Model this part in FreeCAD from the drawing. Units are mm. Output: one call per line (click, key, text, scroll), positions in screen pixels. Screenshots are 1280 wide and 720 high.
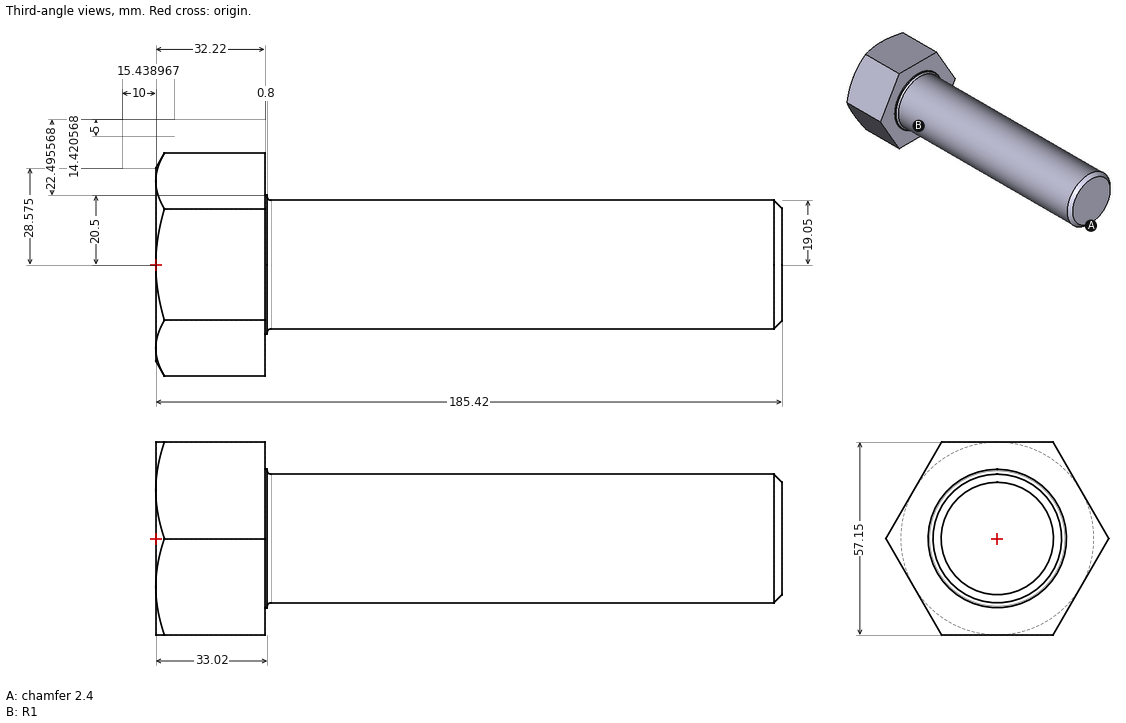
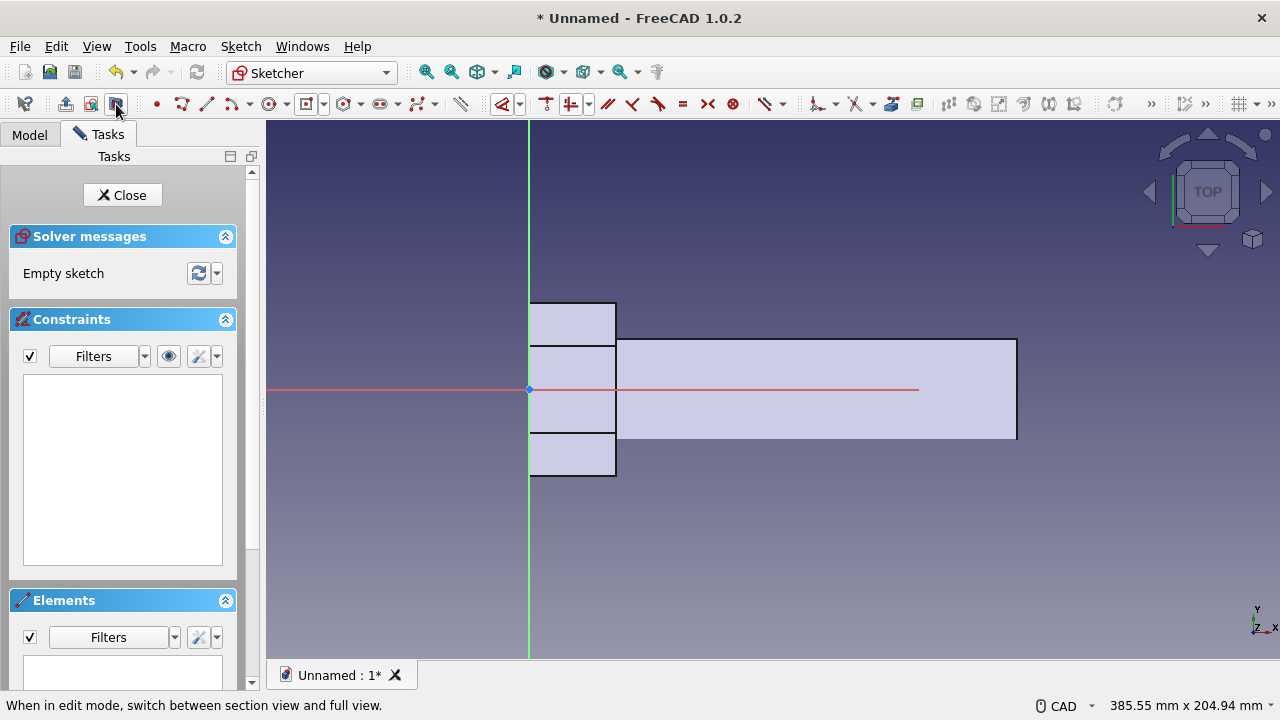
scroll(501, 284, up, 11)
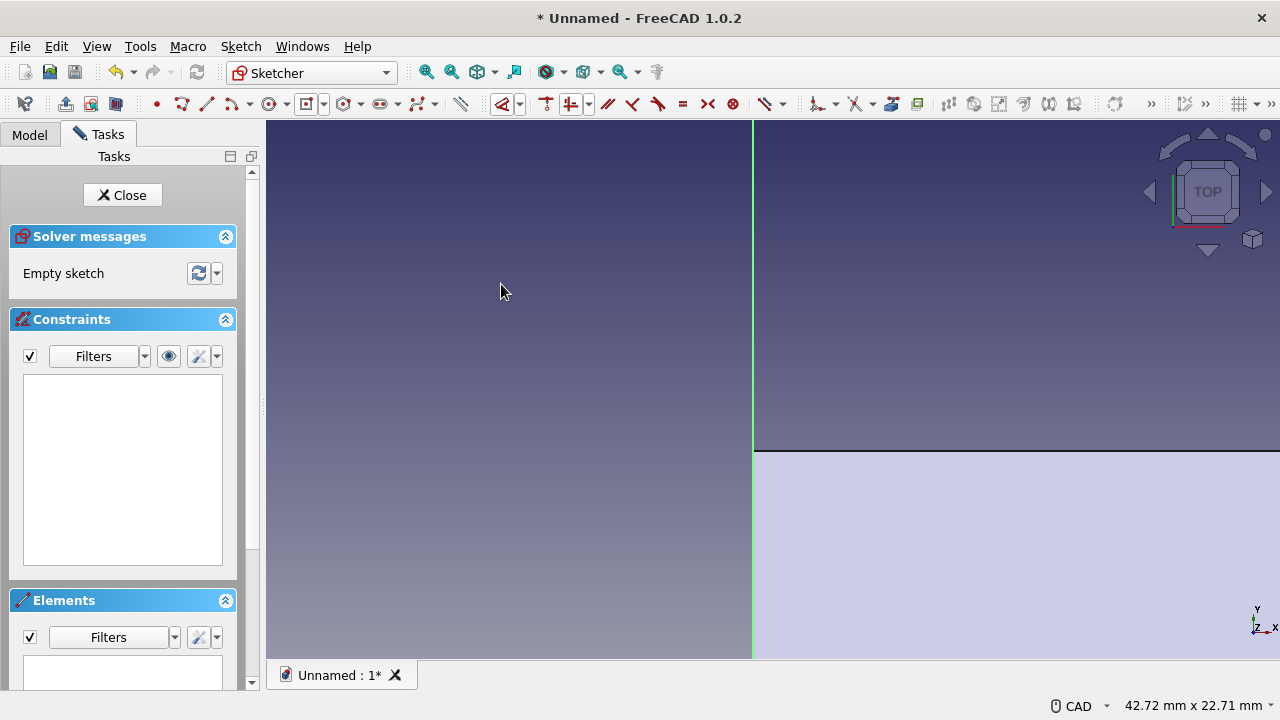
click(182, 104)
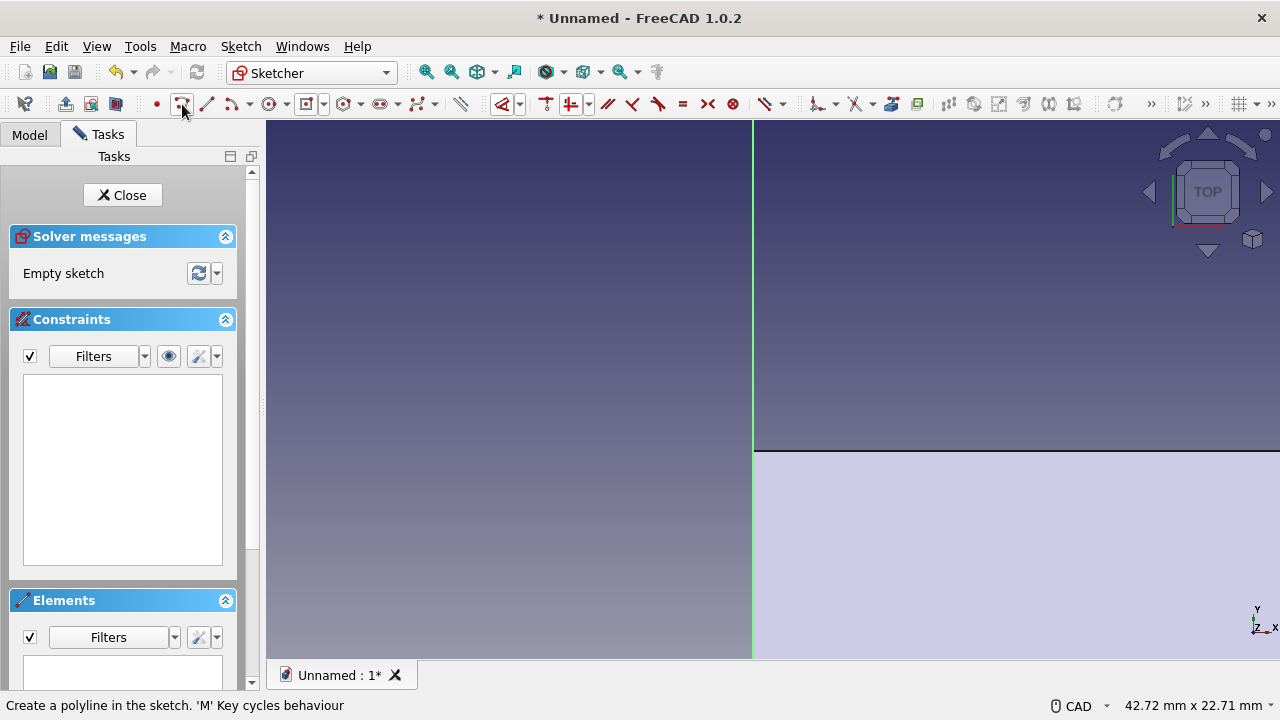
click(753, 555)
click(882, 332)
click(882, 213)
click(516, 213)
click(516, 555)
click(753, 556)
key(Escape)
key(Escape)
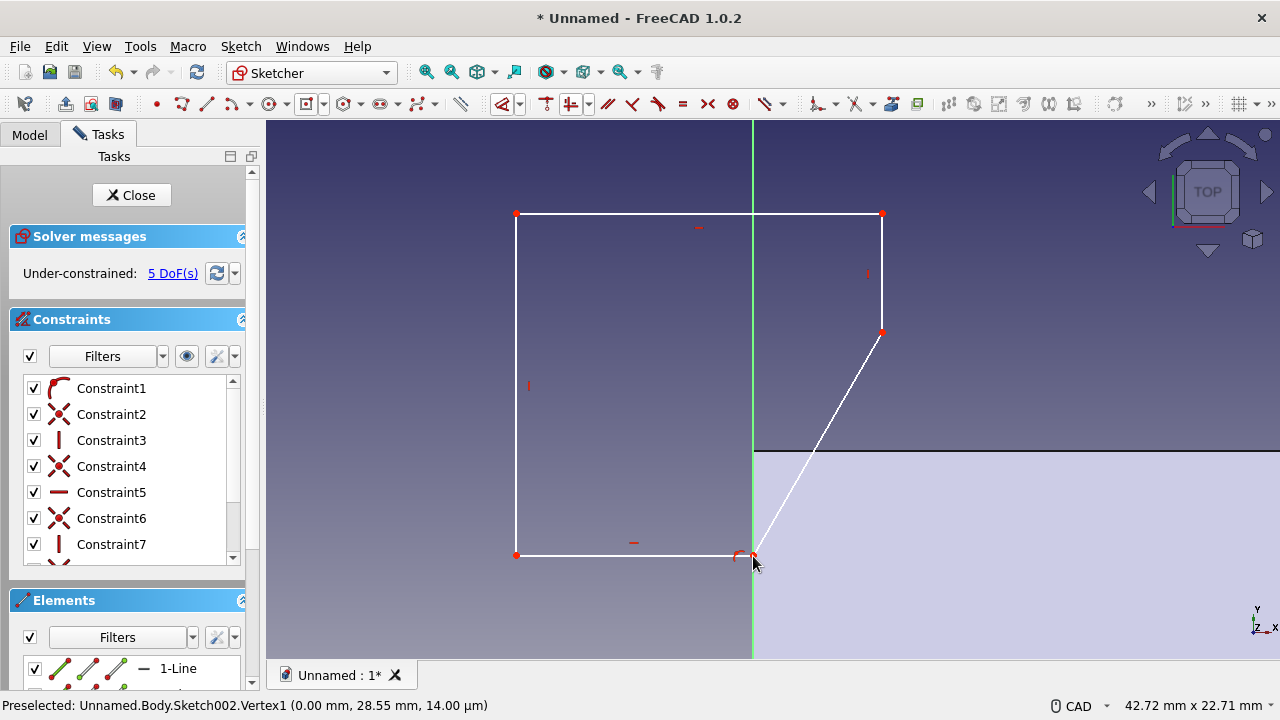
click(882, 297)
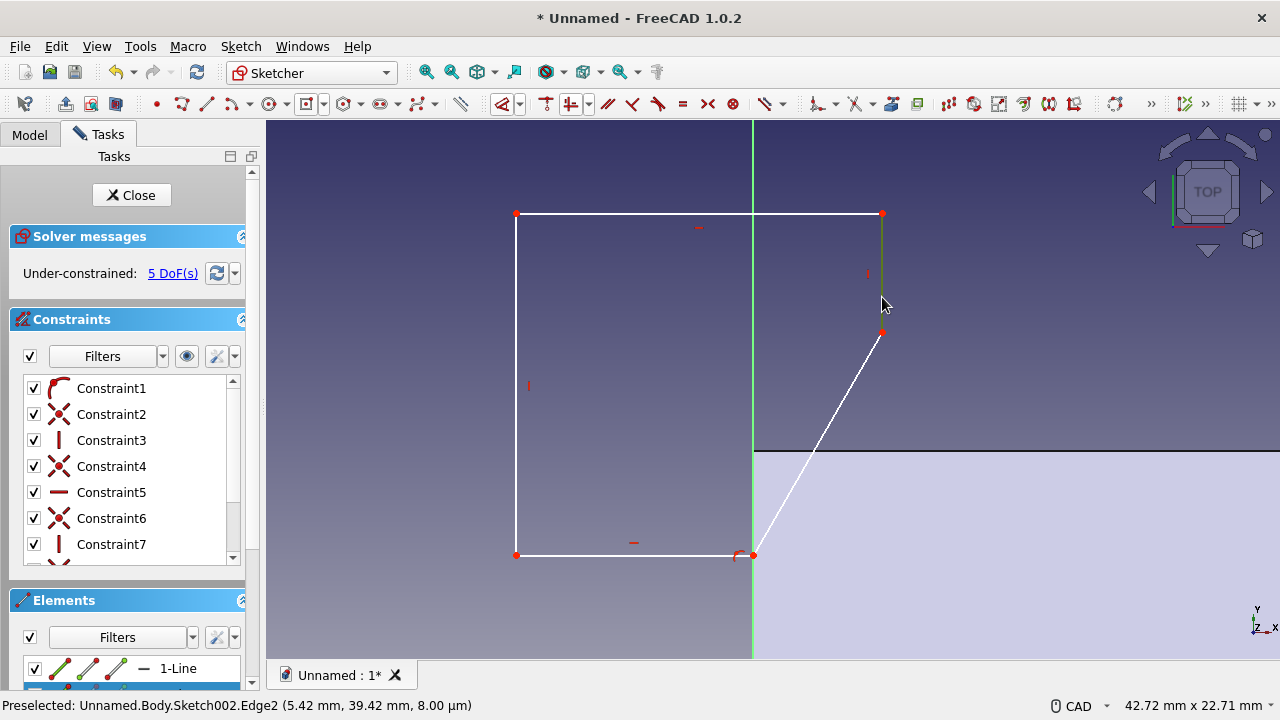
key(i)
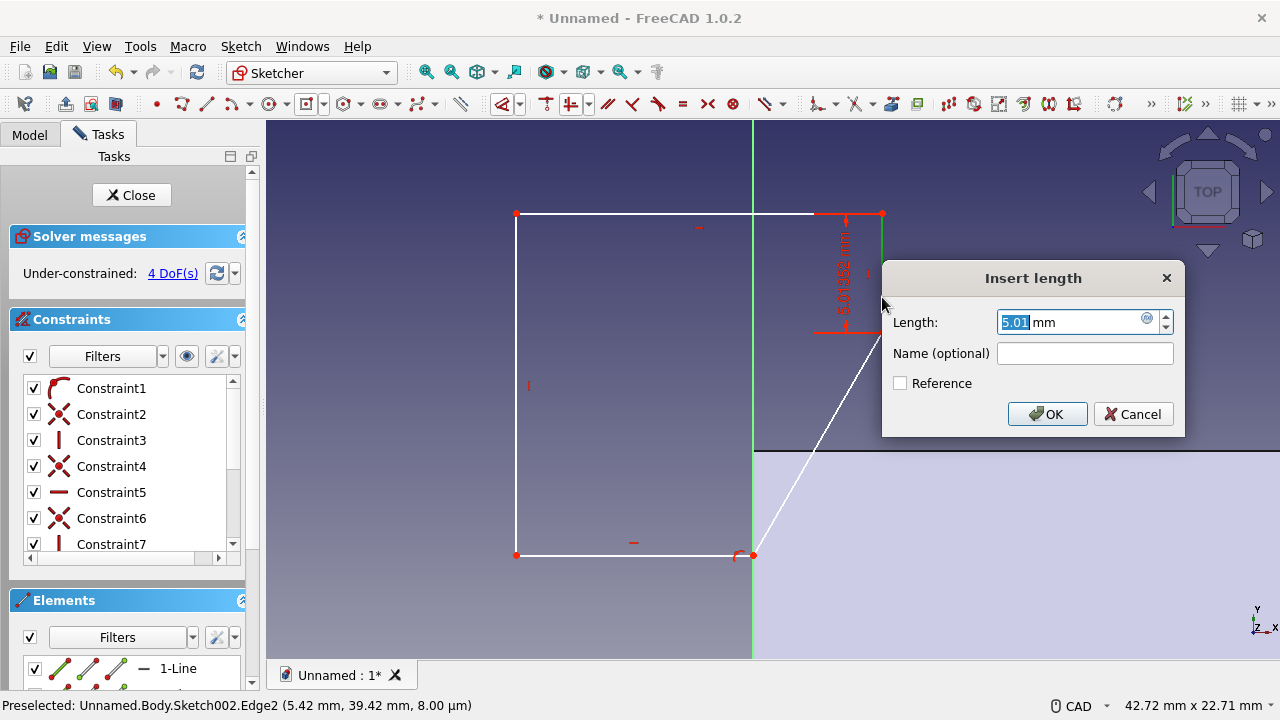
text(5)
key(Return)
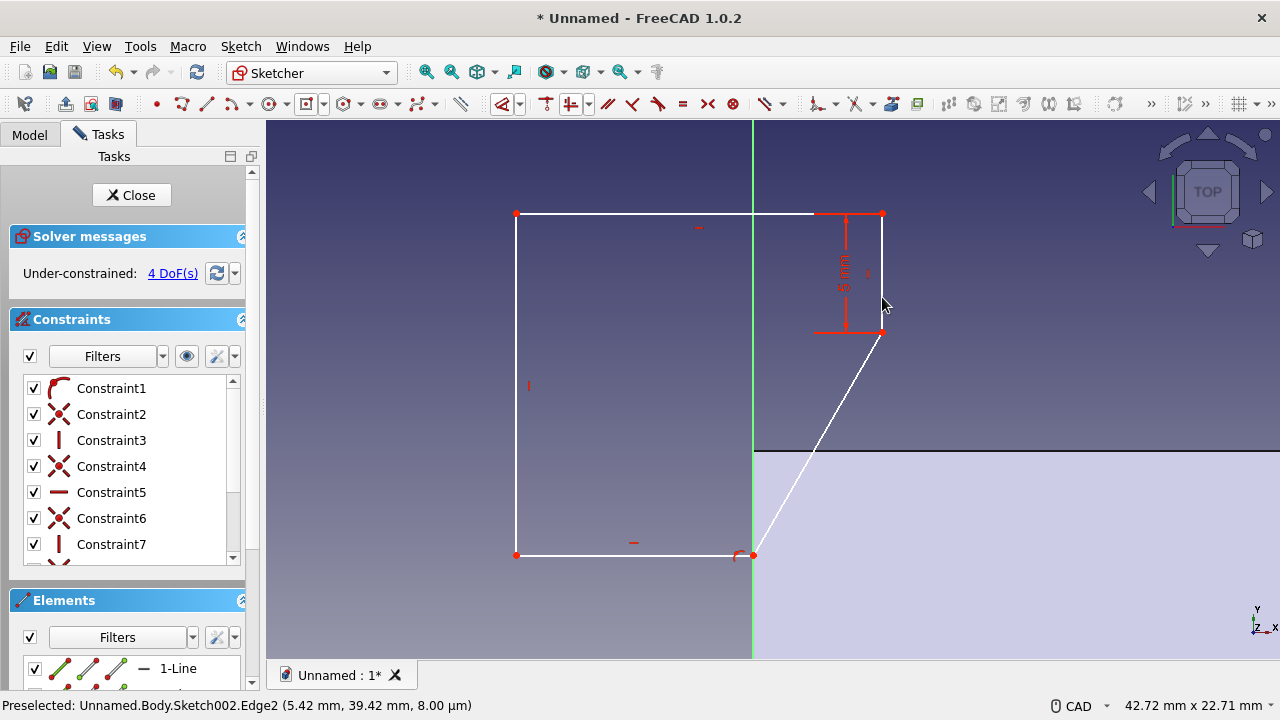
click(587, 556)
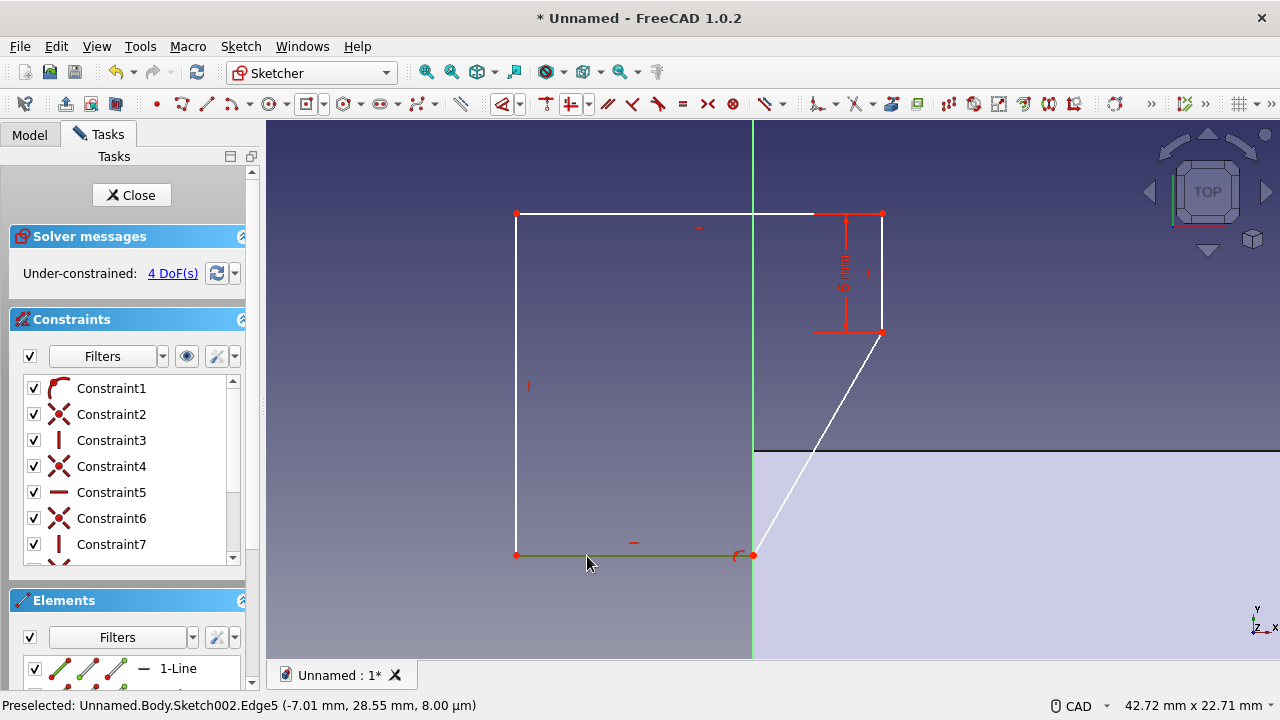
key(l)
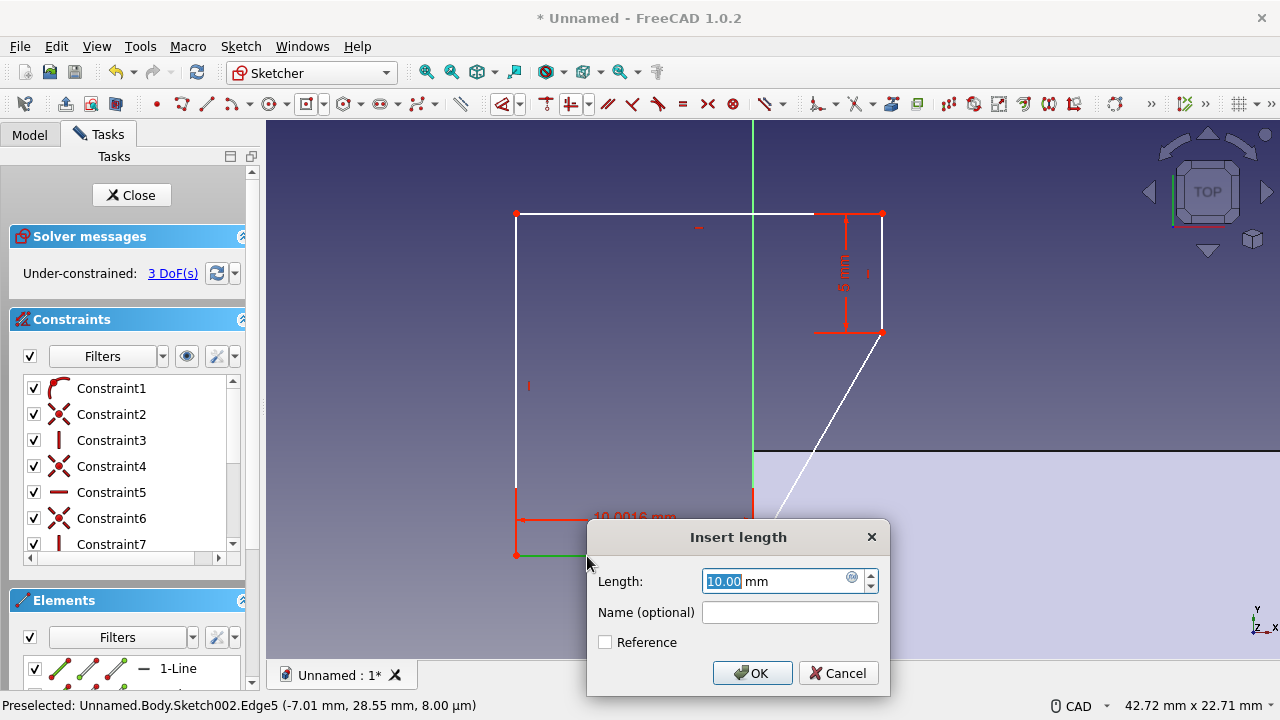
text(10)
key(Return)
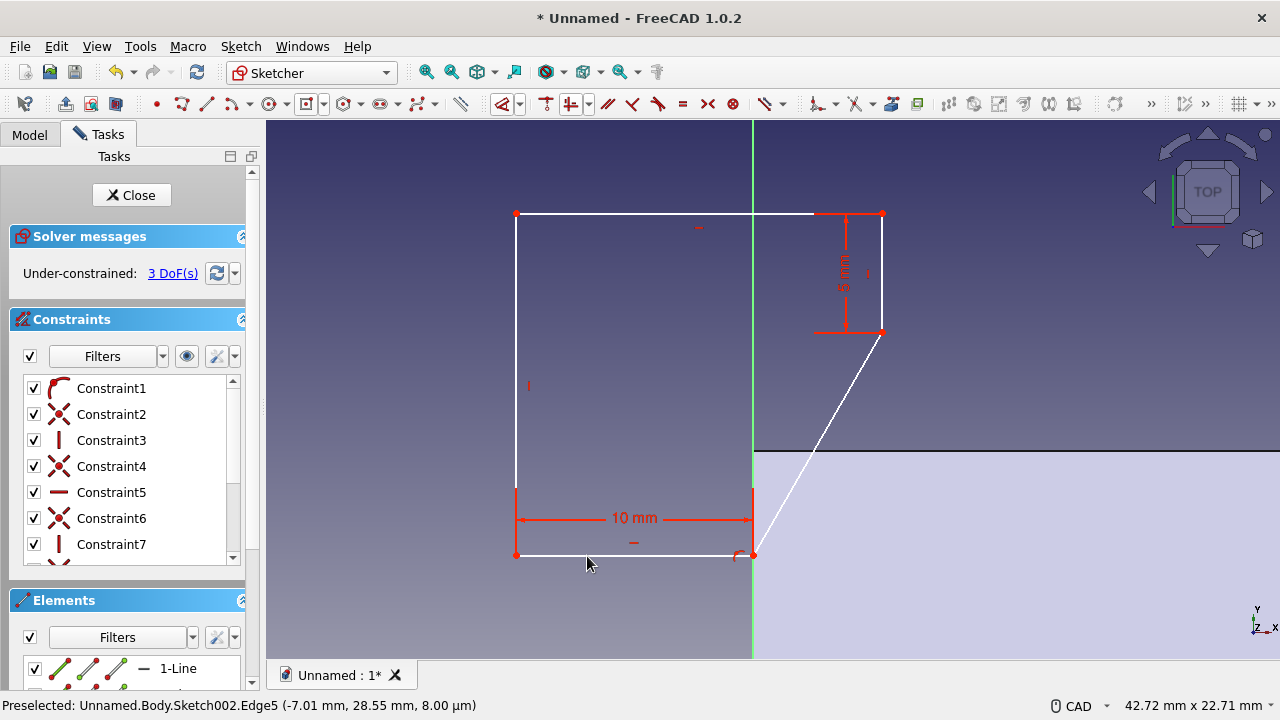
click(753, 556)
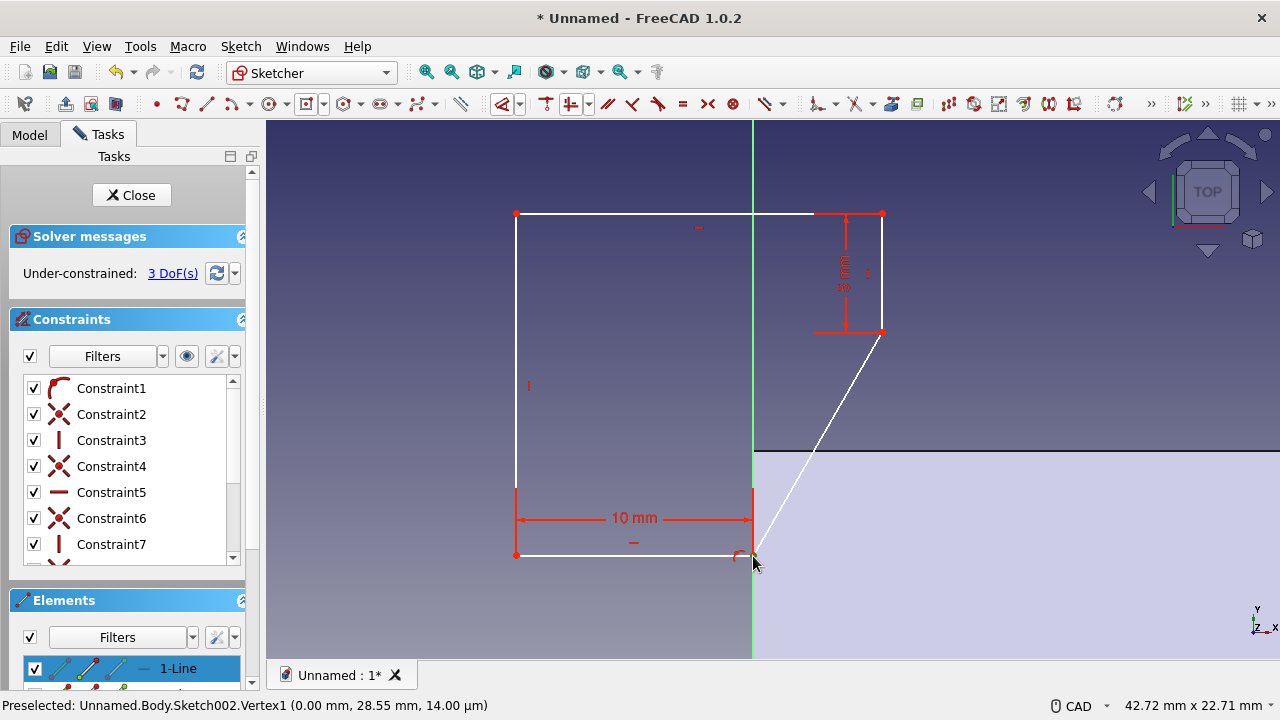
key(i)